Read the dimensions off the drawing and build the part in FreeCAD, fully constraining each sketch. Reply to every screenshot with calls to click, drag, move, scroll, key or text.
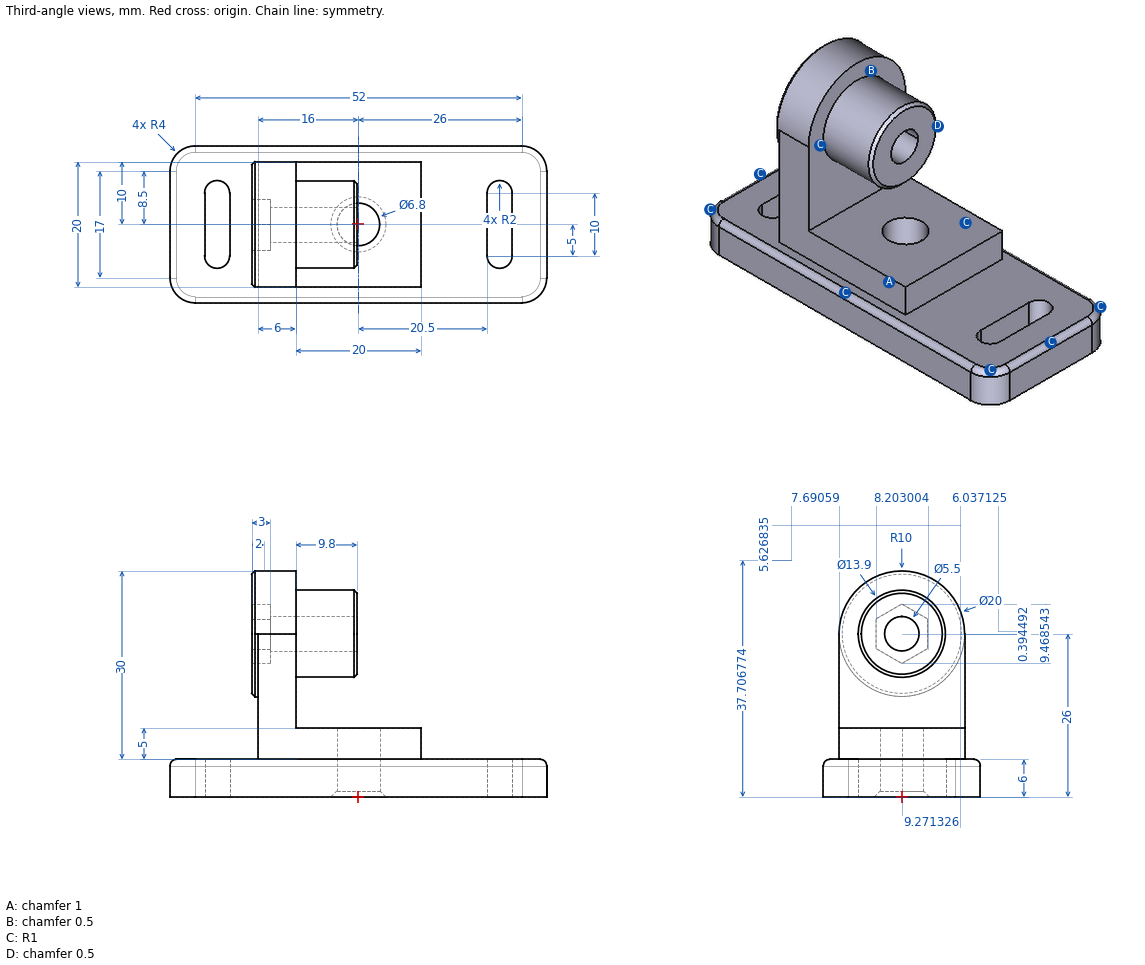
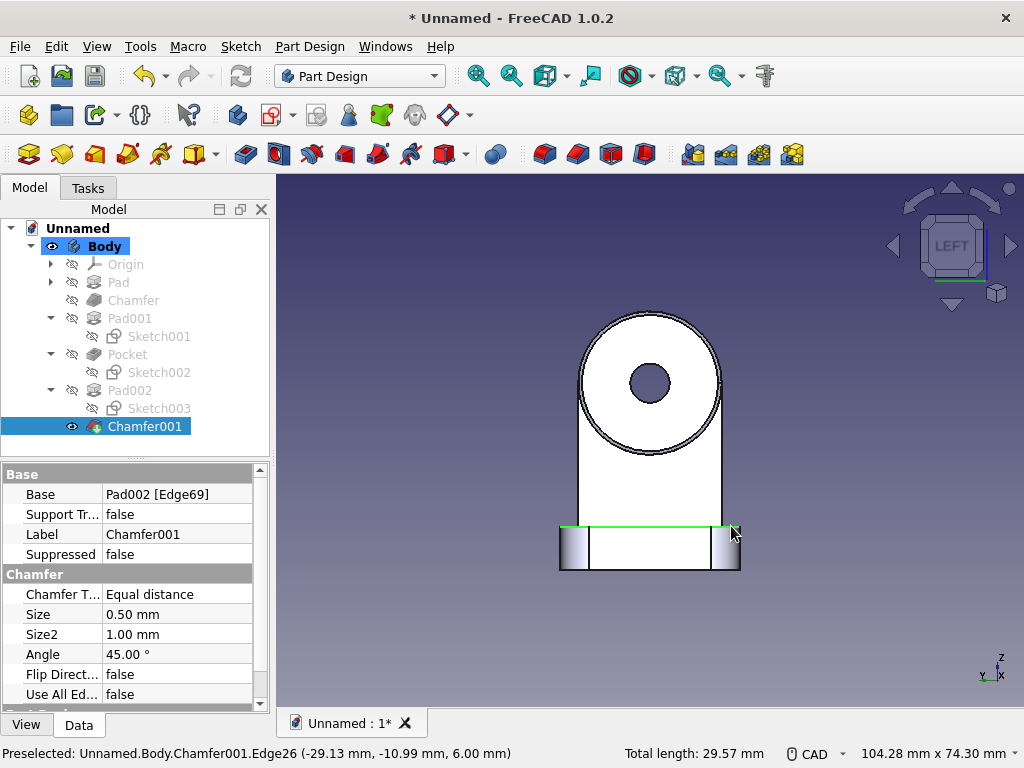
key(0)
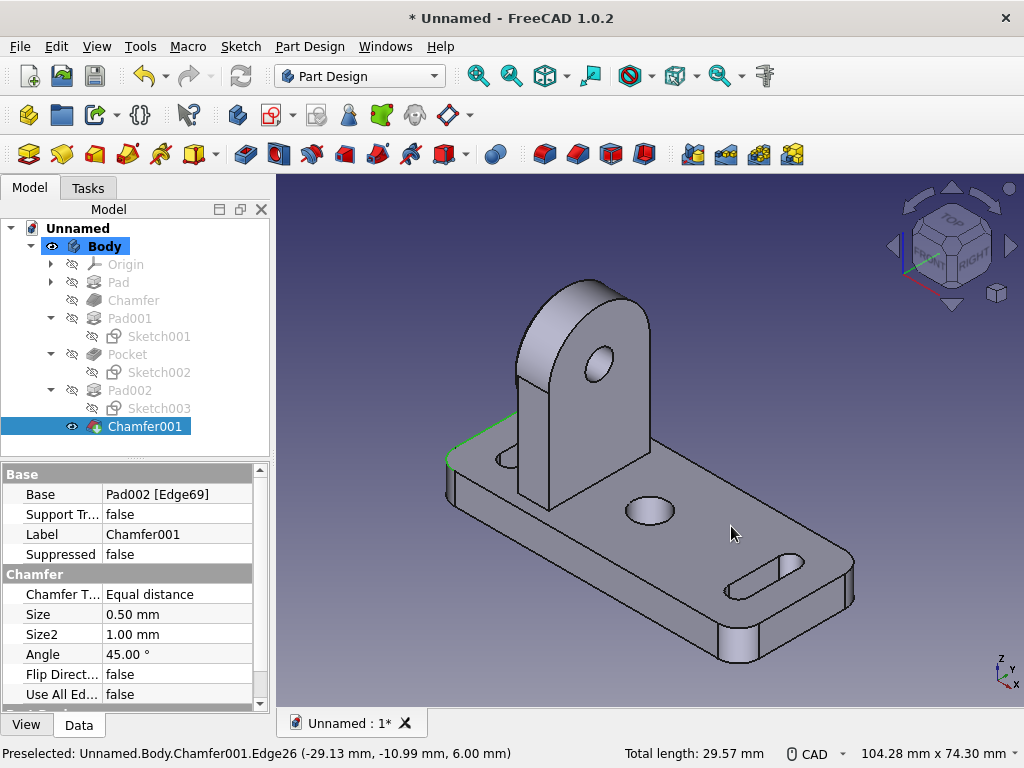
click(739, 627, ctrl)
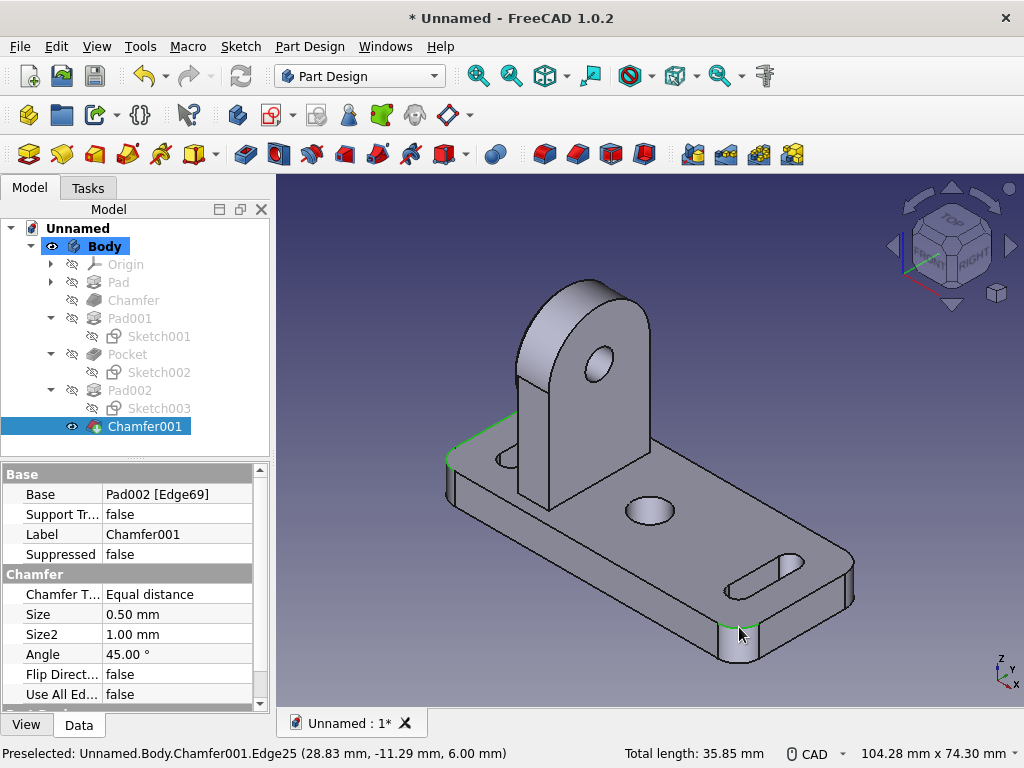
click(802, 598, ctrl)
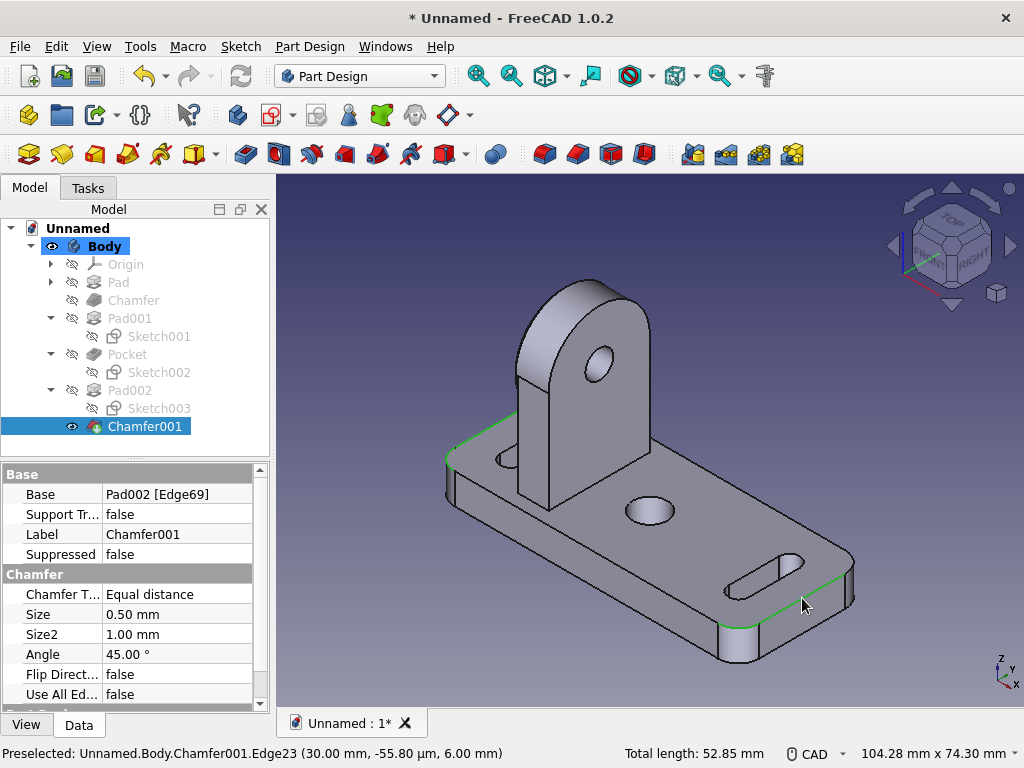
click(854, 561, ctrl)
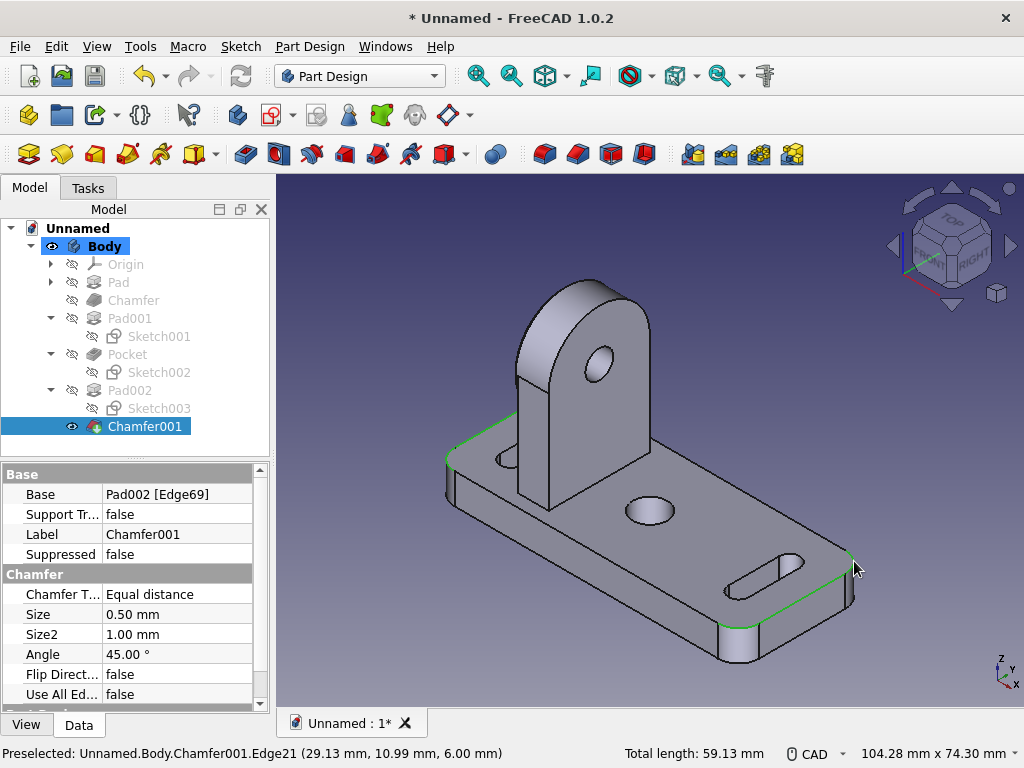
click(587, 546, ctrl)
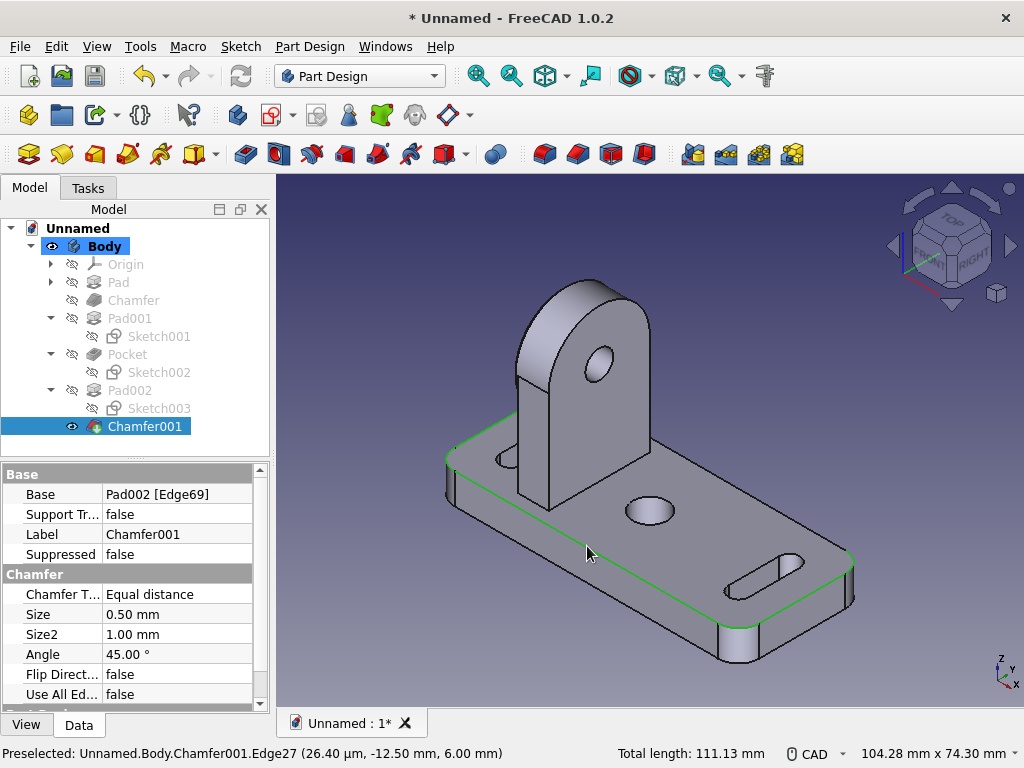
key(2)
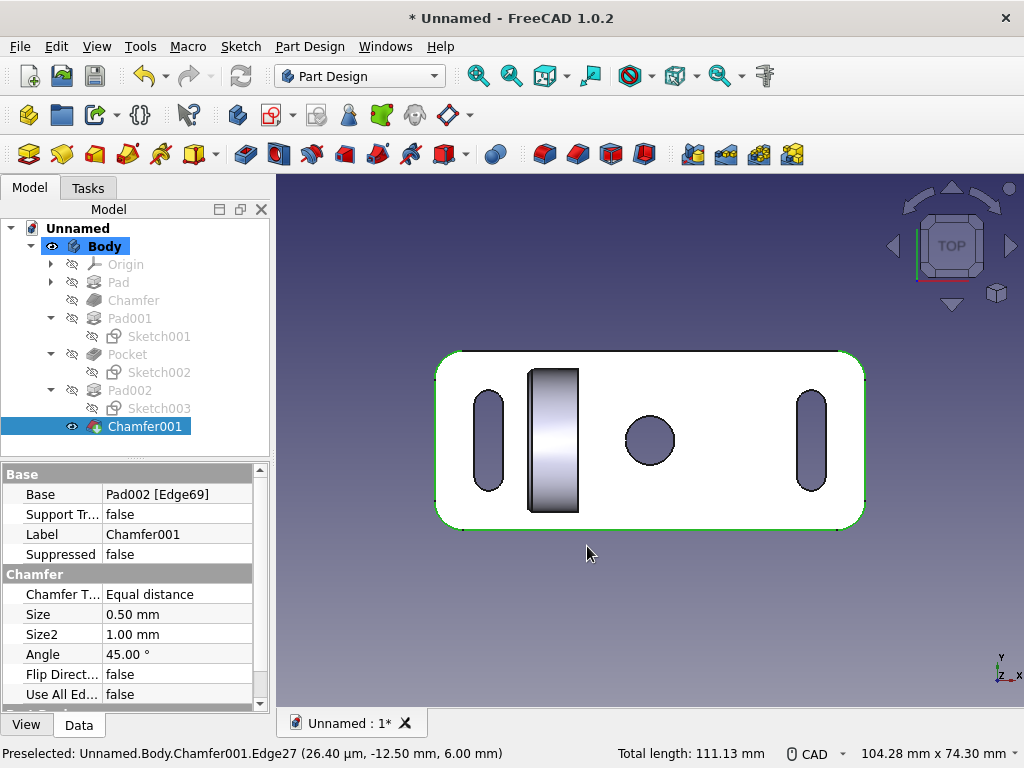
click(650, 350, ctrl)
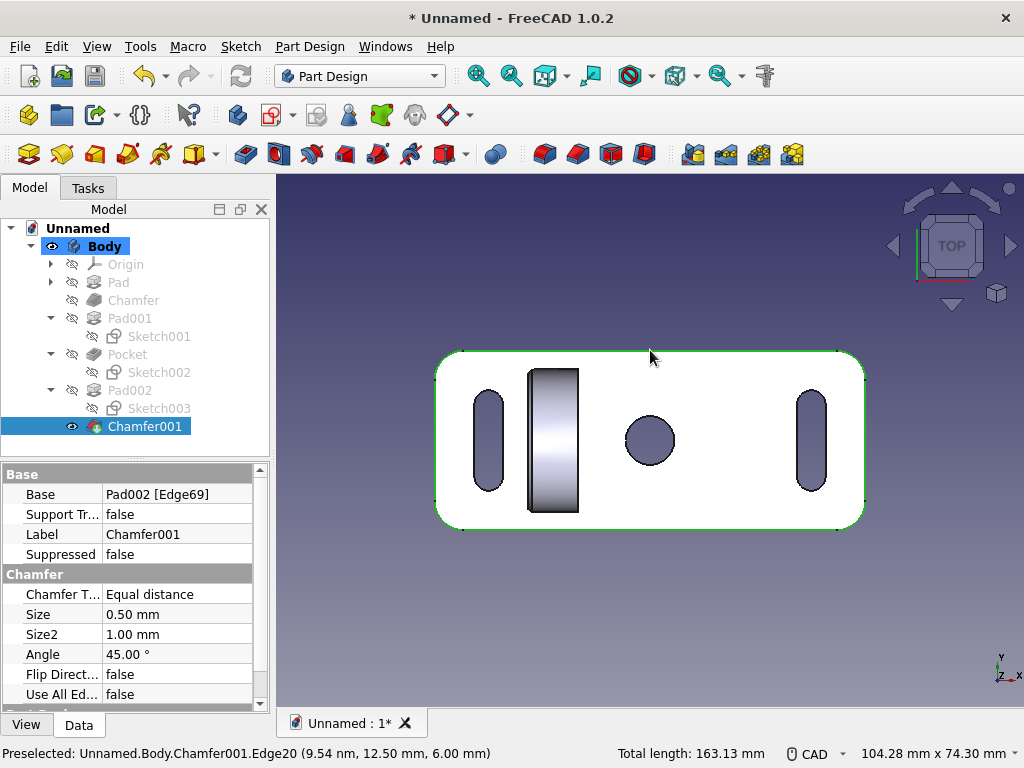
click(545, 154)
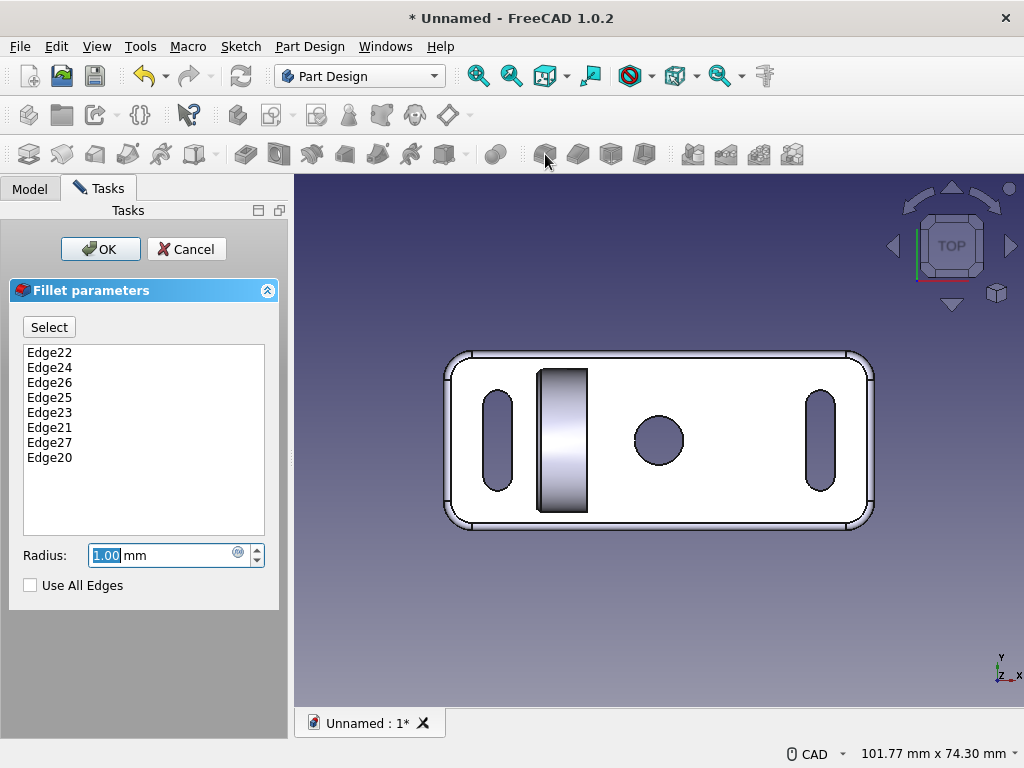
text(1)
key(Tab)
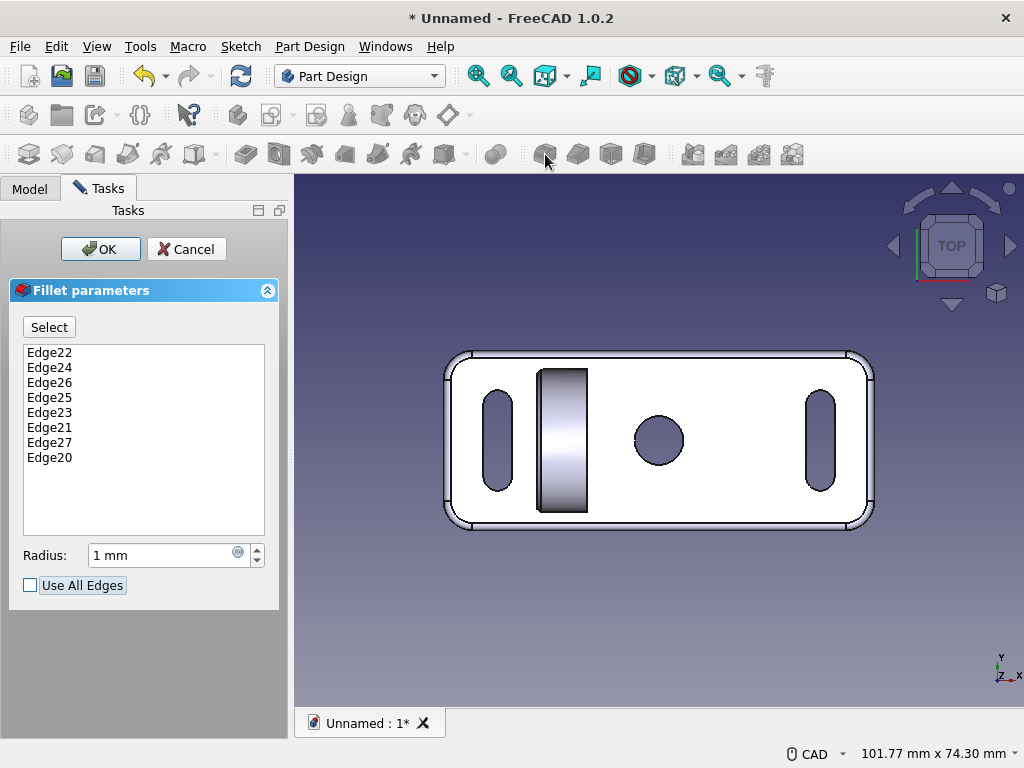
click(101, 249)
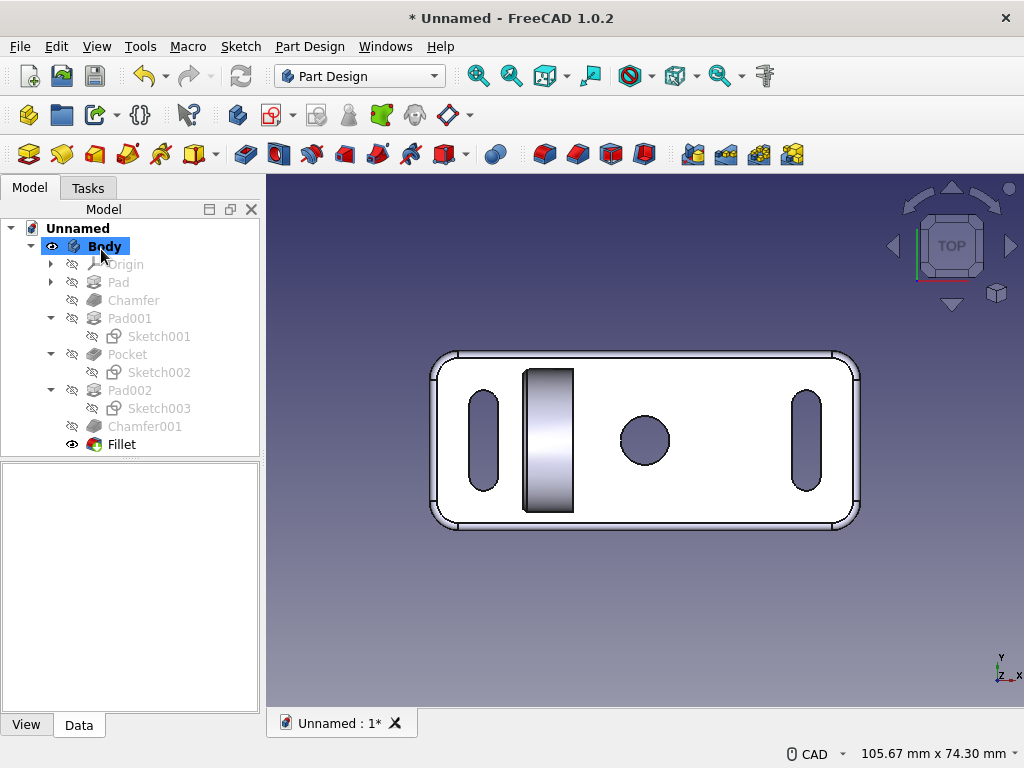
click(704, 463)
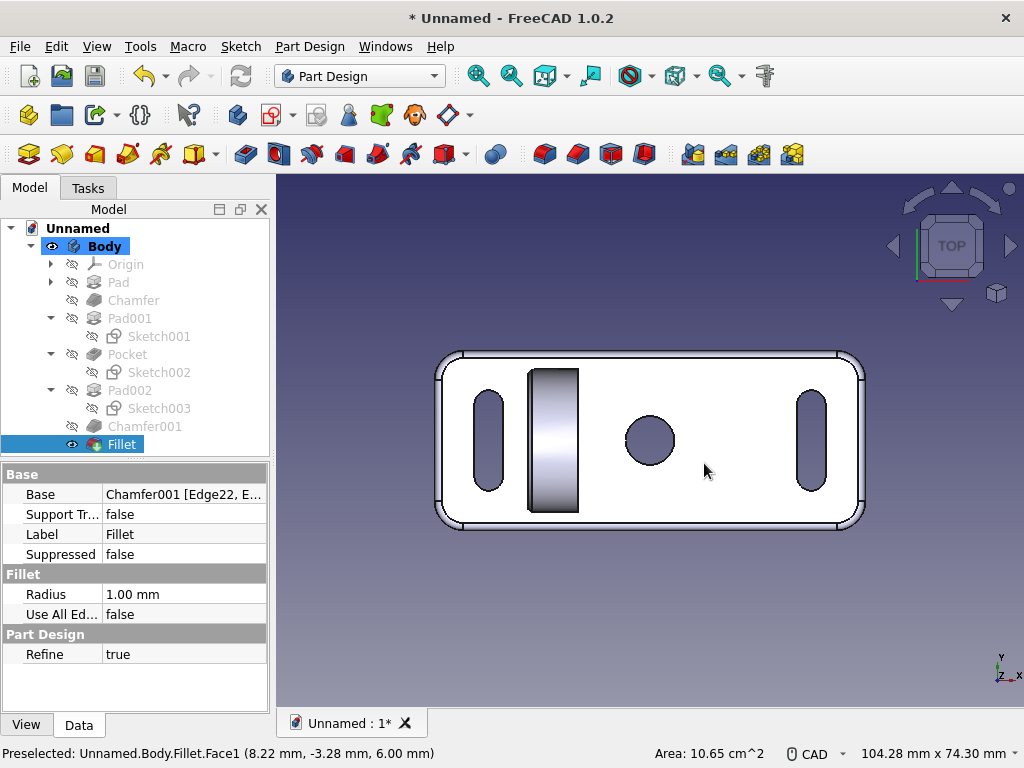
click(270, 116)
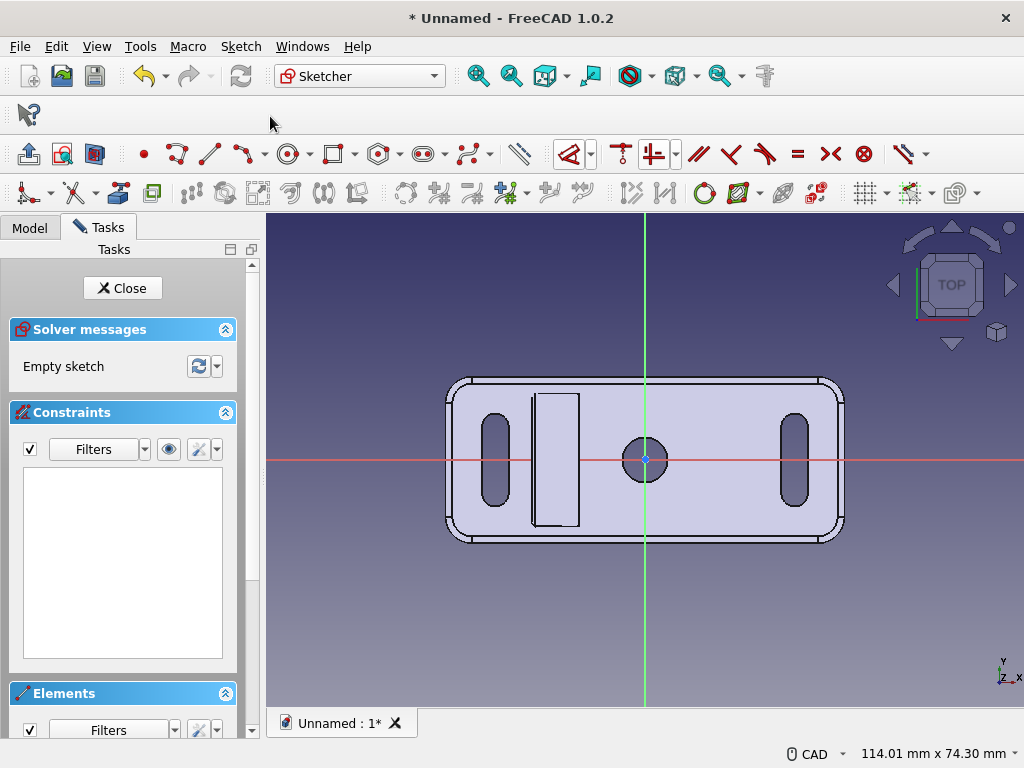
click(95, 154)